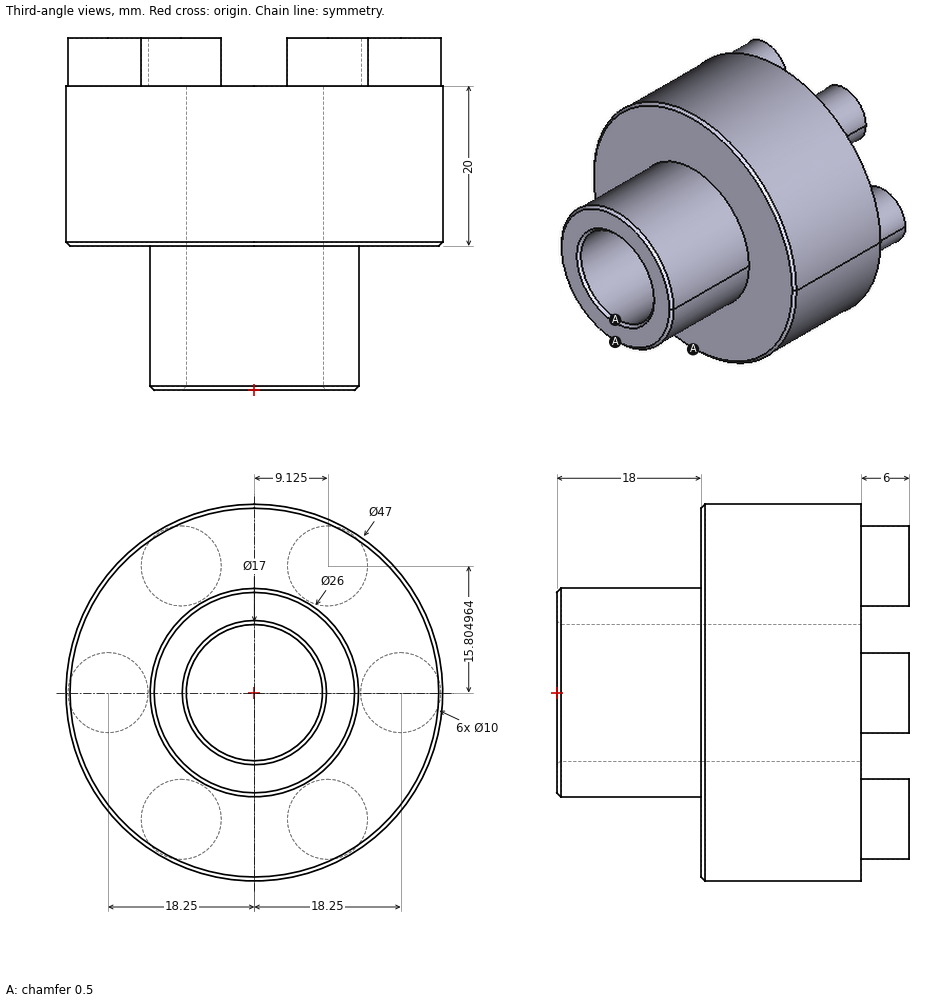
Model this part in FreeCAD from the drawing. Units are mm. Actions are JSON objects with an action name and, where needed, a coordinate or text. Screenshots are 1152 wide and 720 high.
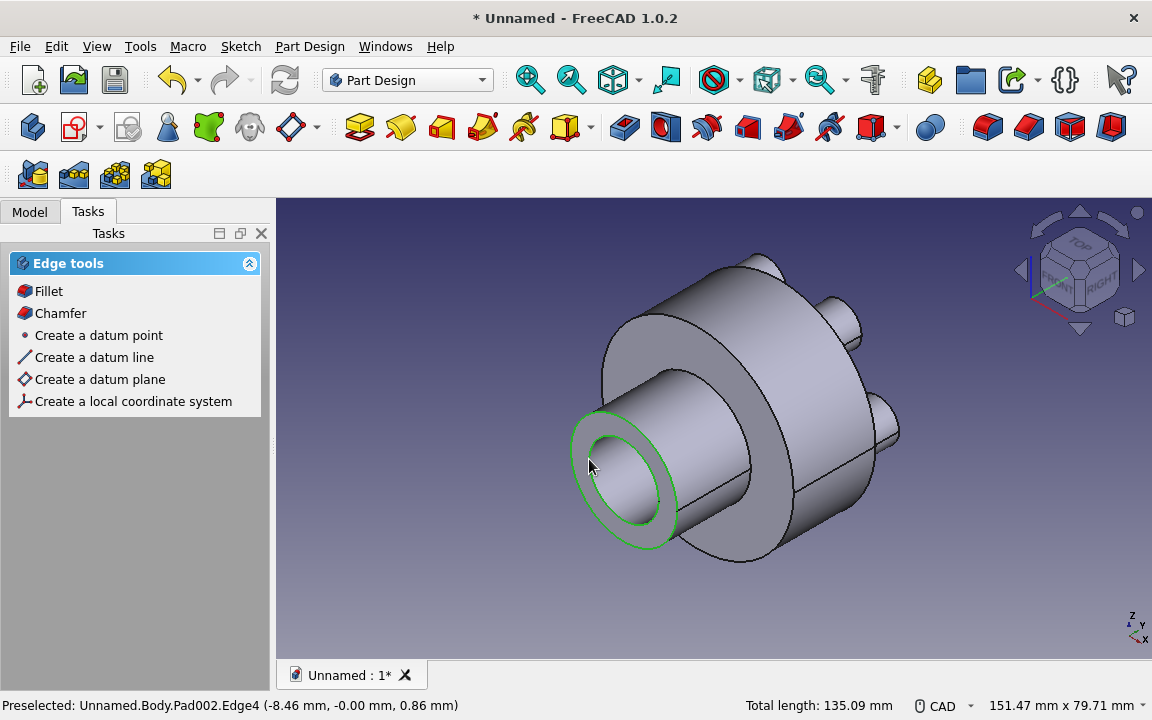
{"action": "left_click", "coordinate": [668, 314], "text": "ctrl"}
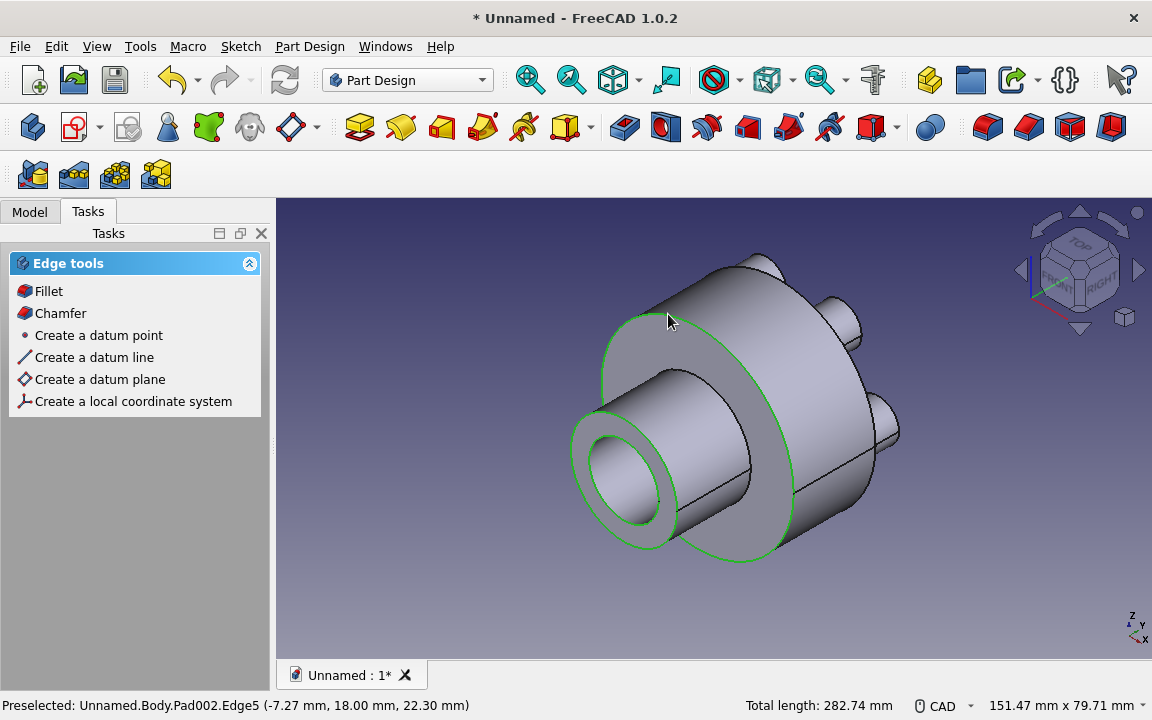
{"action": "left_click", "coordinate": [1029, 128]}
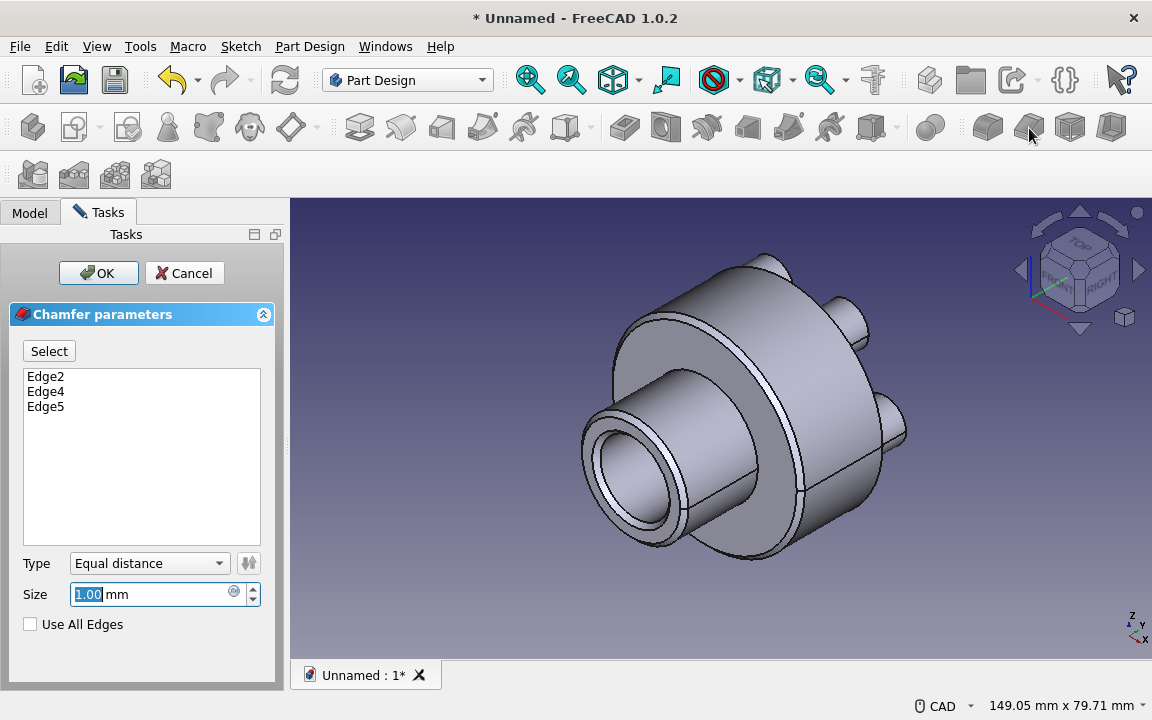
{"action": "type", "text": "0.5"}
{"action": "key", "text": "Tab"}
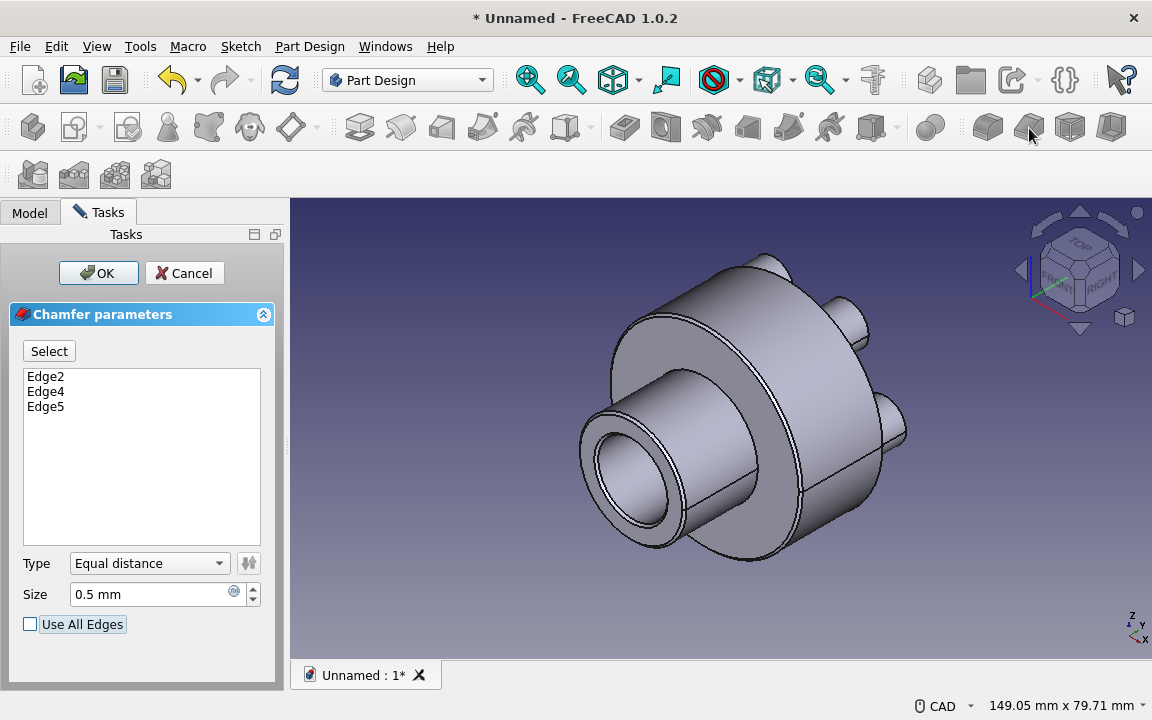
{"action": "left_click", "coordinate": [99, 273]}